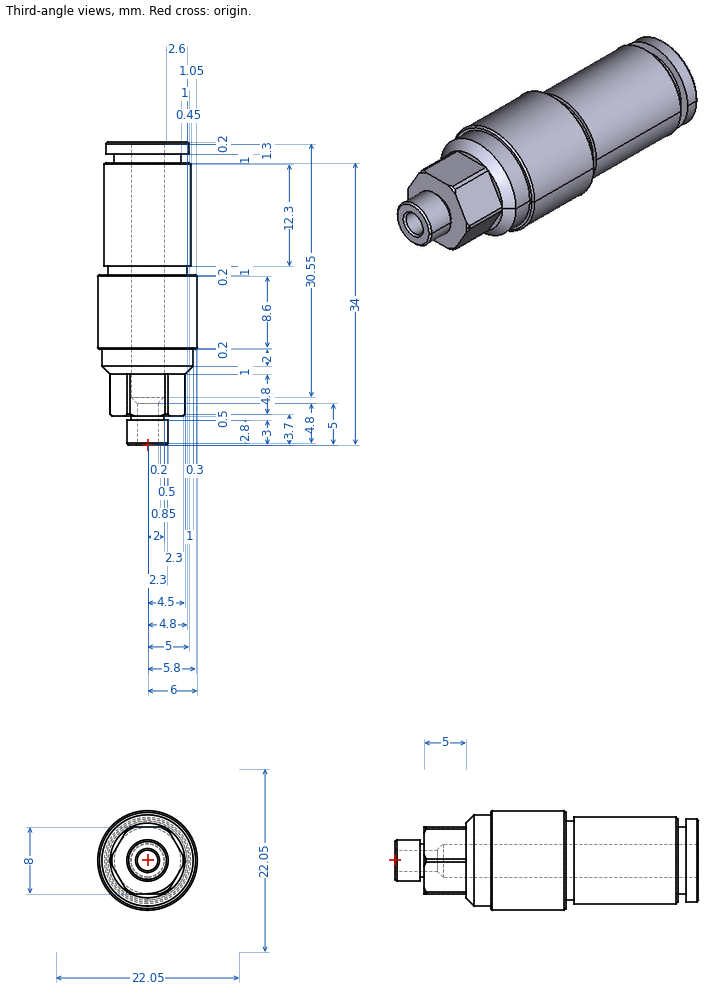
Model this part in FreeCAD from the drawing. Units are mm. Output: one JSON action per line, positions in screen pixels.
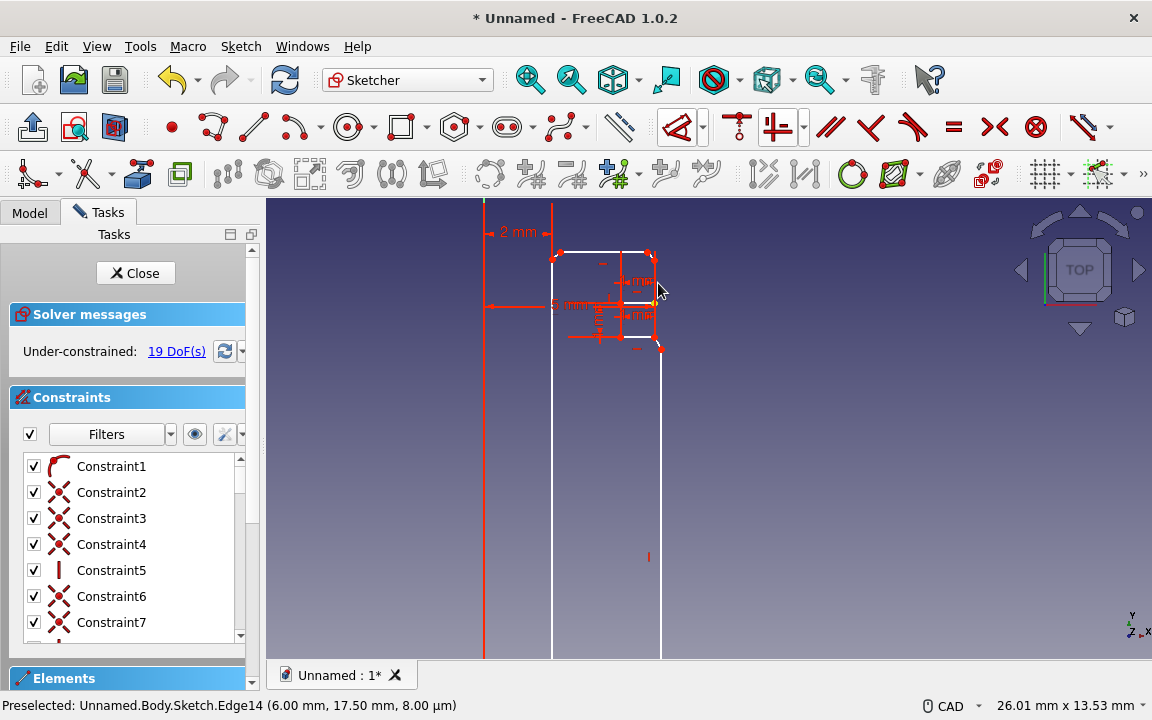
{"action": "left_click", "coordinate": [655, 290]}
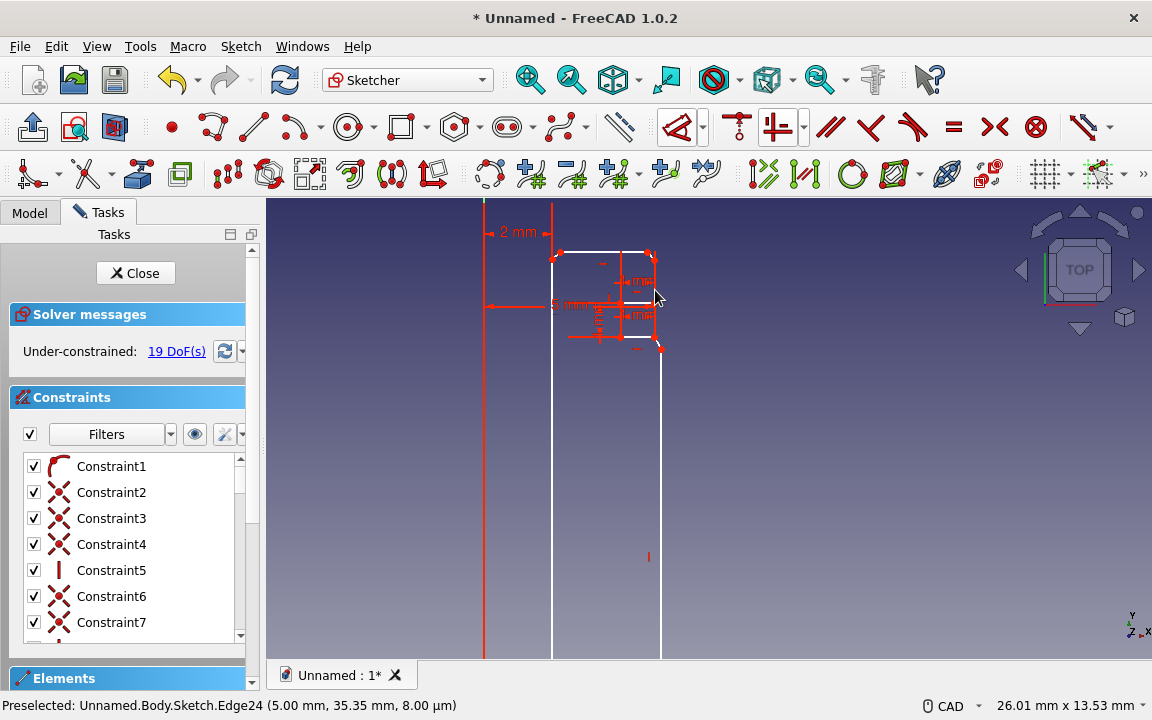
{"action": "key", "text": "i"}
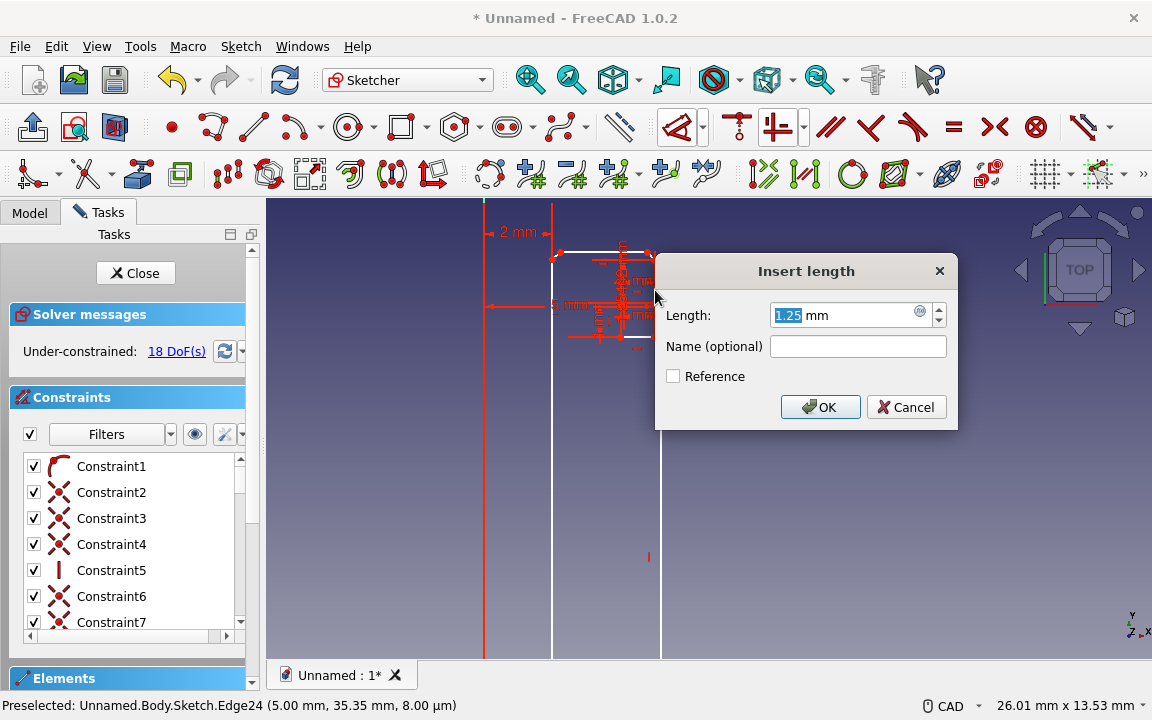
{"action": "type", "text": "1.3"}
{"action": "key", "text": "Return"}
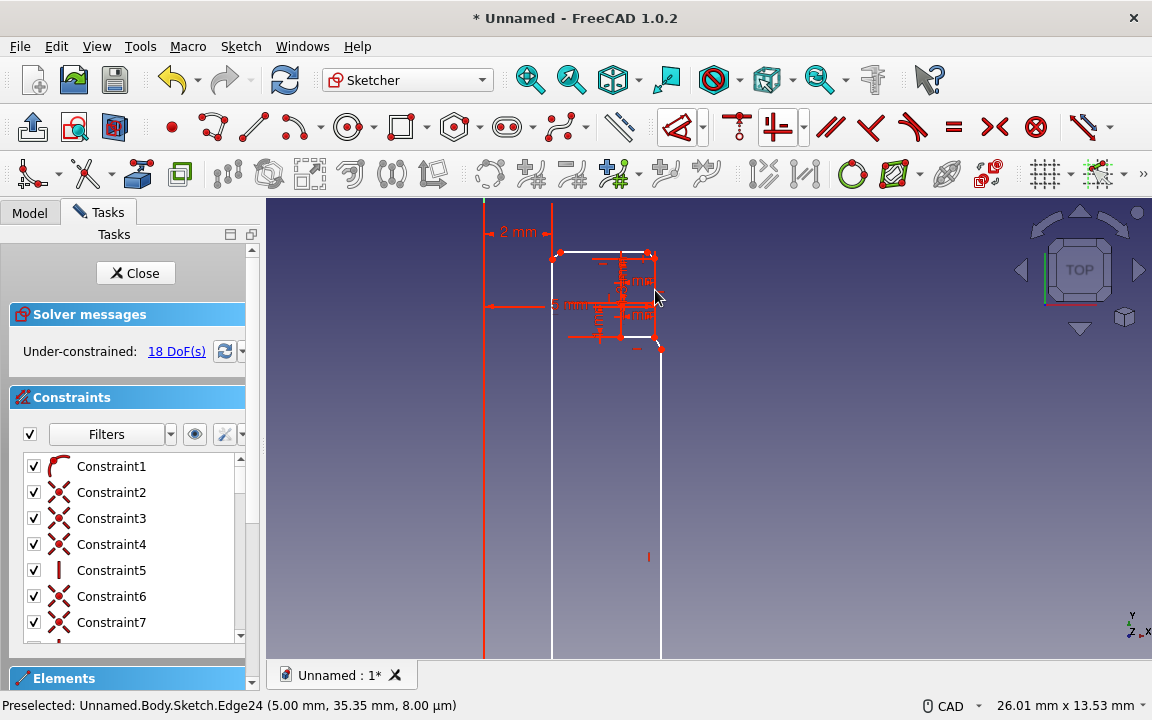
{"action": "left_click", "coordinate": [621, 252]}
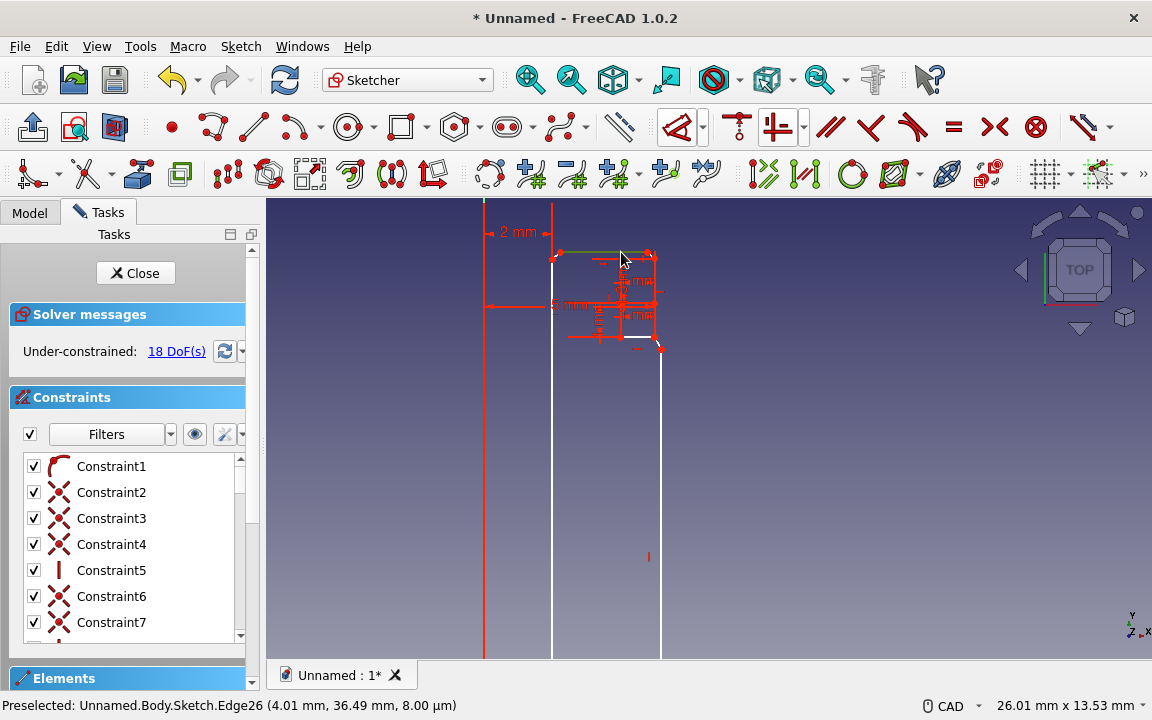
{"action": "key", "text": "l"}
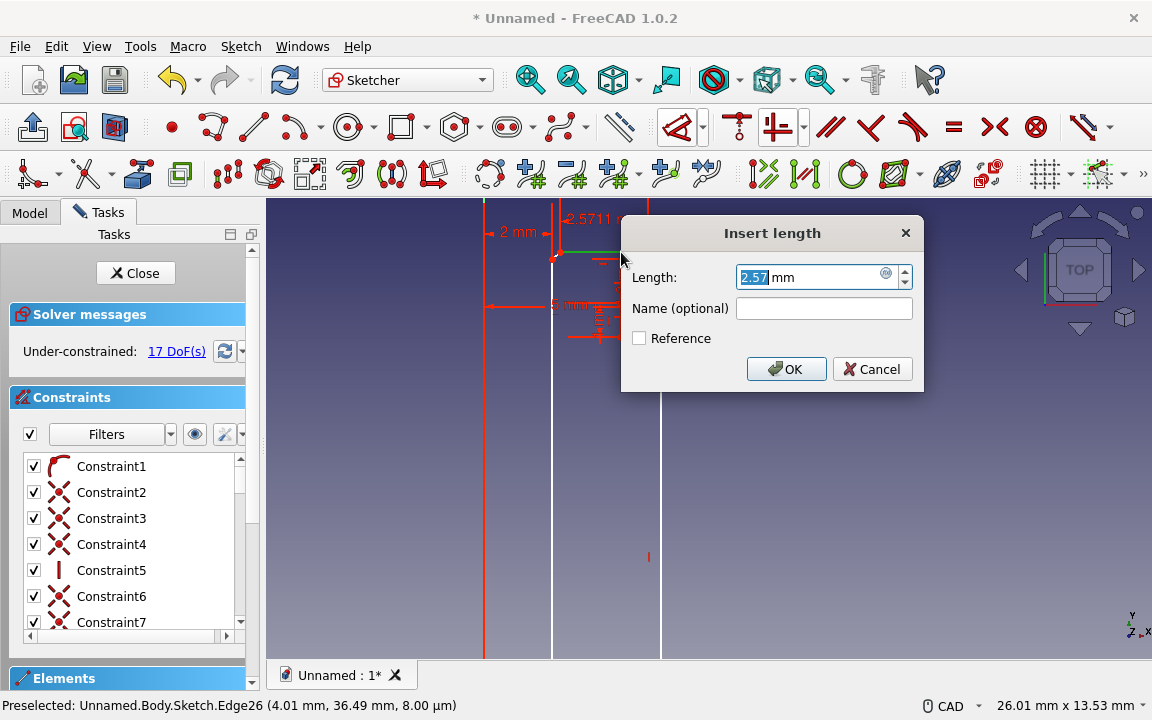
{"action": "type", "text": "2.6"}
{"action": "key", "text": "Return"}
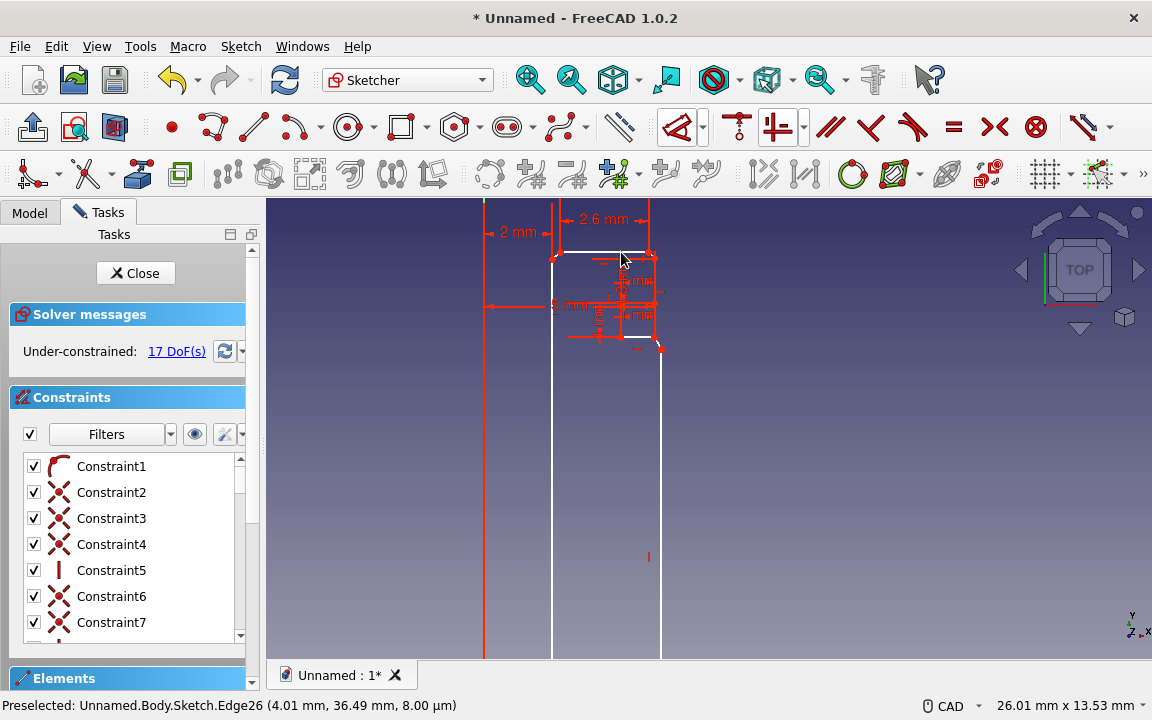
{"action": "scroll", "coordinate": [658, 283], "scroll_direction": "down", "scroll_amount": 7}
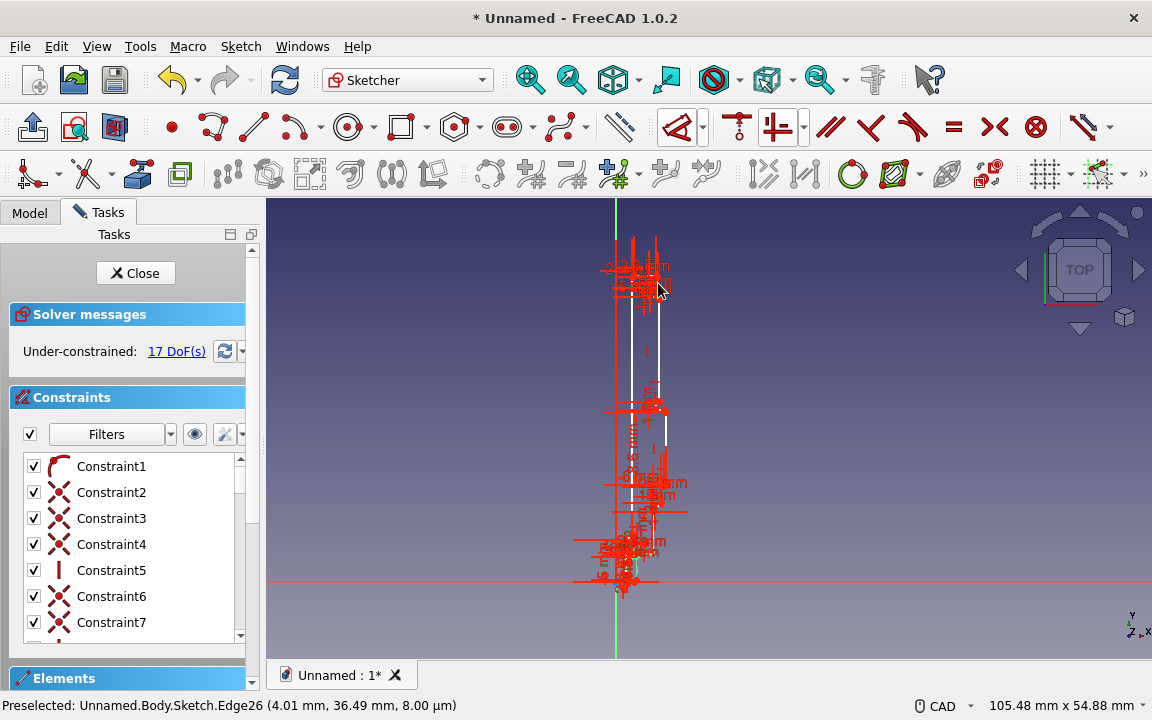
{"action": "scroll", "coordinate": [626, 552], "scroll_direction": "up", "scroll_amount": 4}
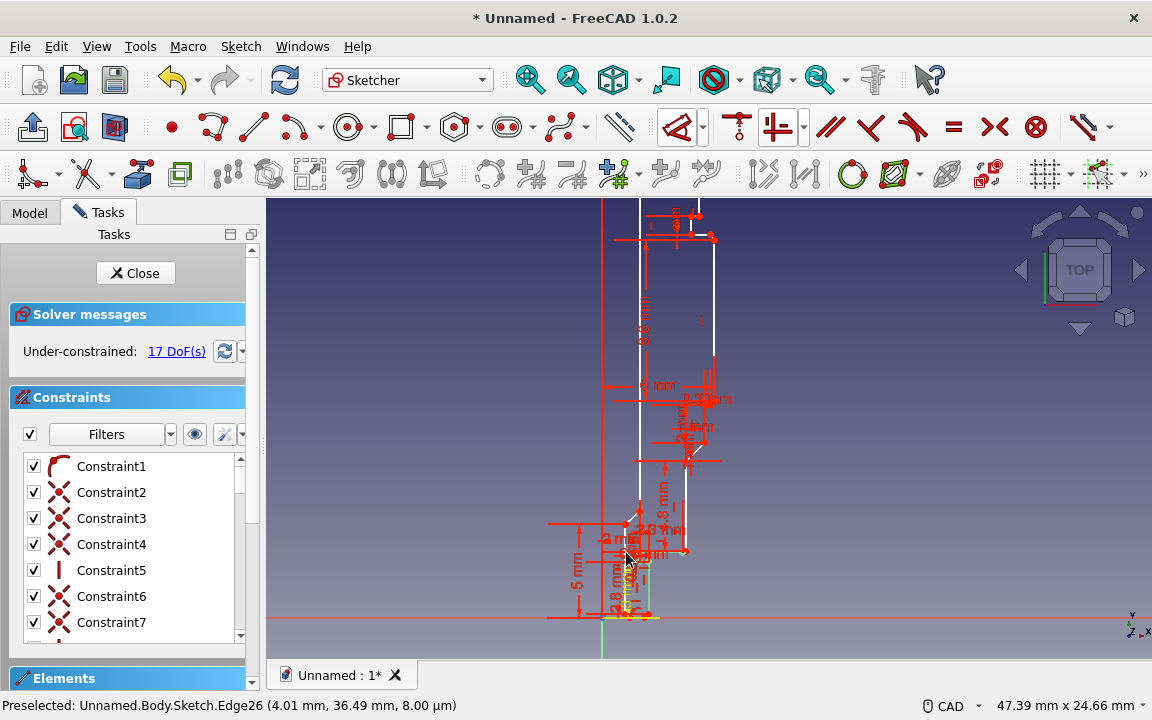
{"action": "scroll", "coordinate": [625, 551], "scroll_direction": "up", "scroll_amount": 4}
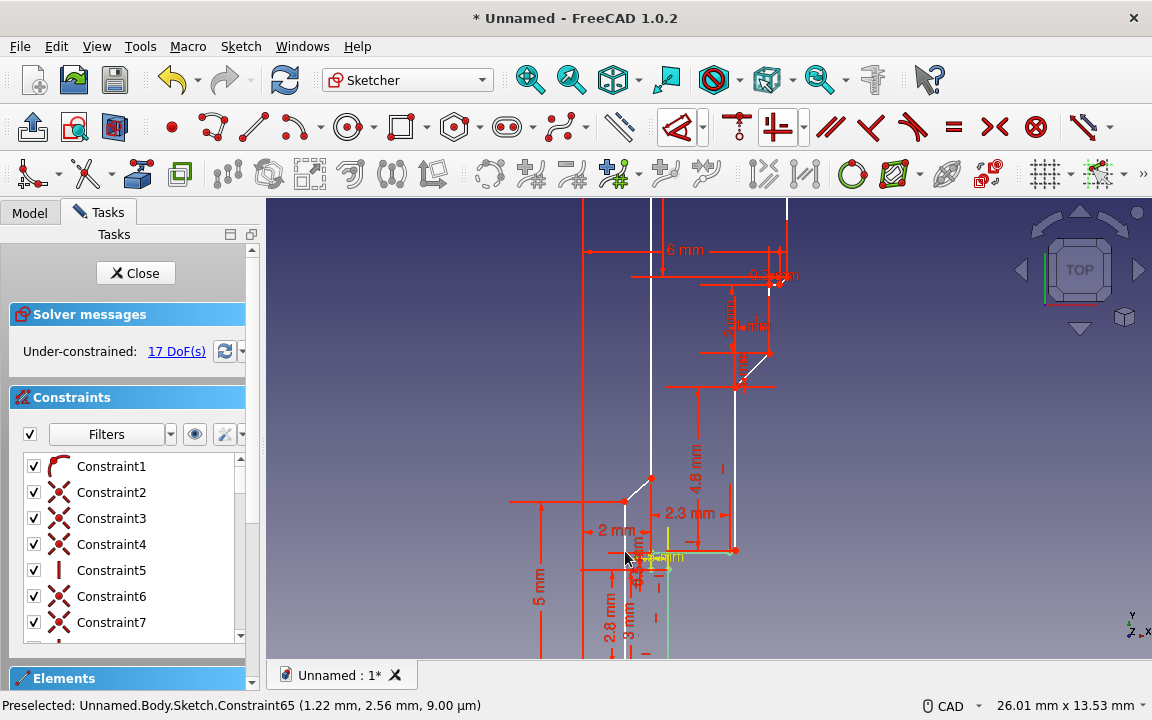
{"action": "left_click", "coordinate": [625, 551]}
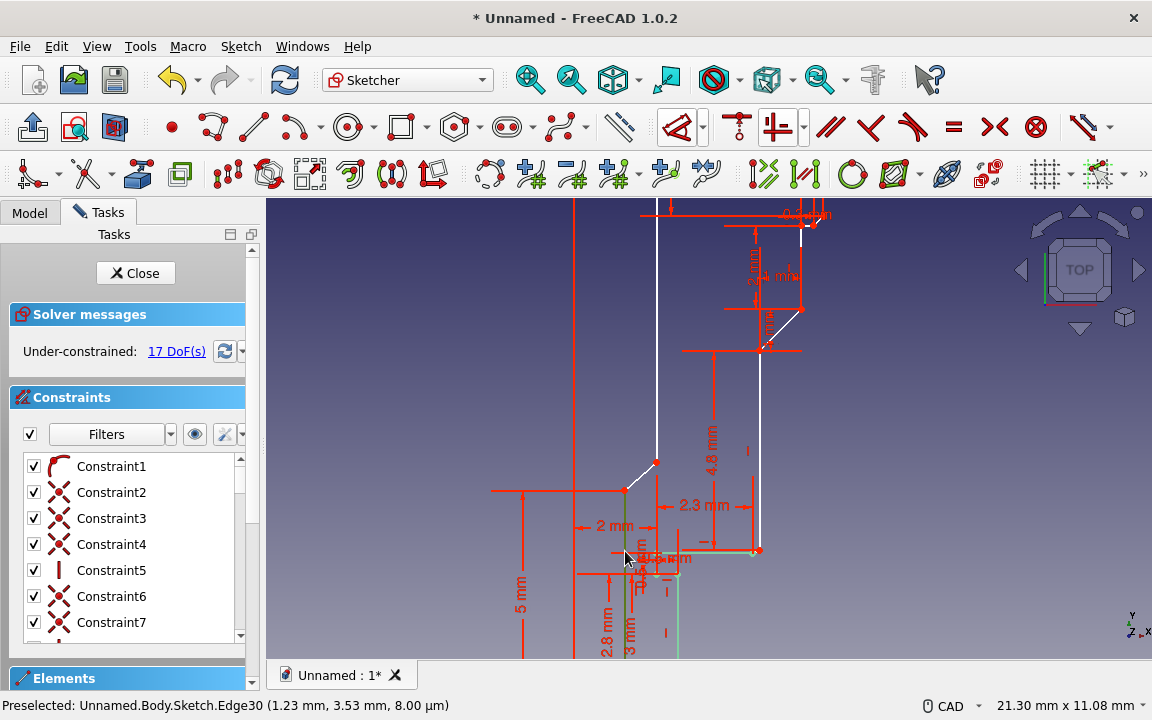
{"action": "left_click", "coordinate": [702, 128]}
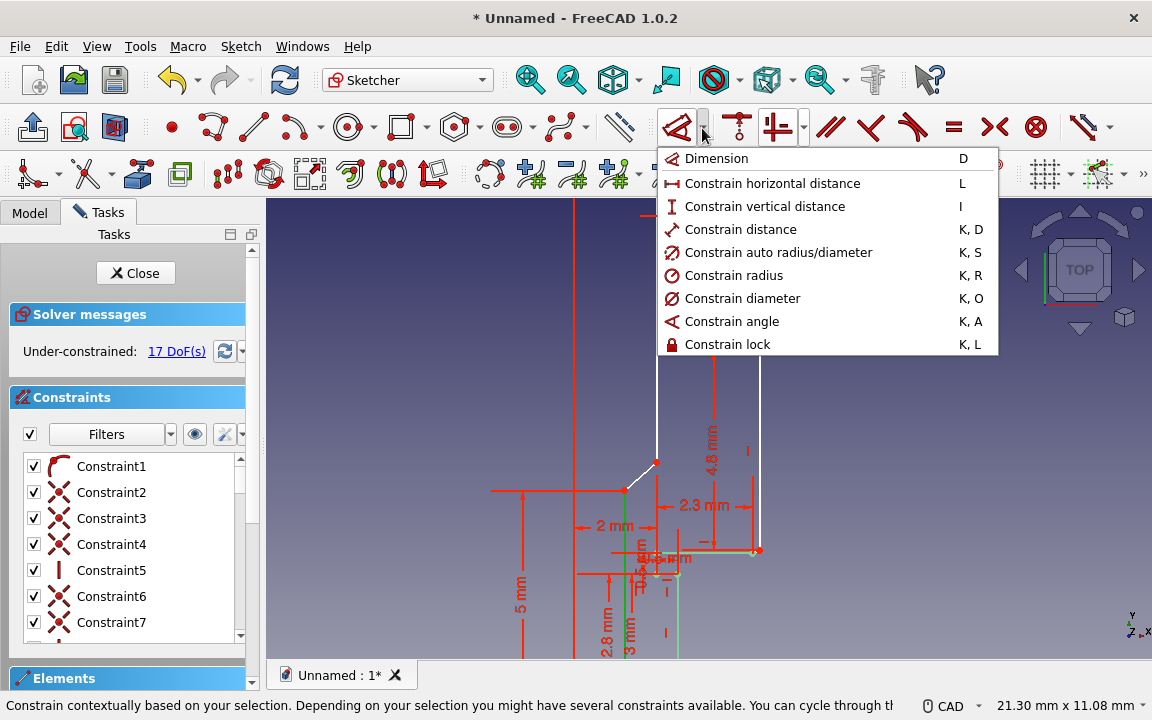
{"action": "left_click", "coordinate": [828, 206]}